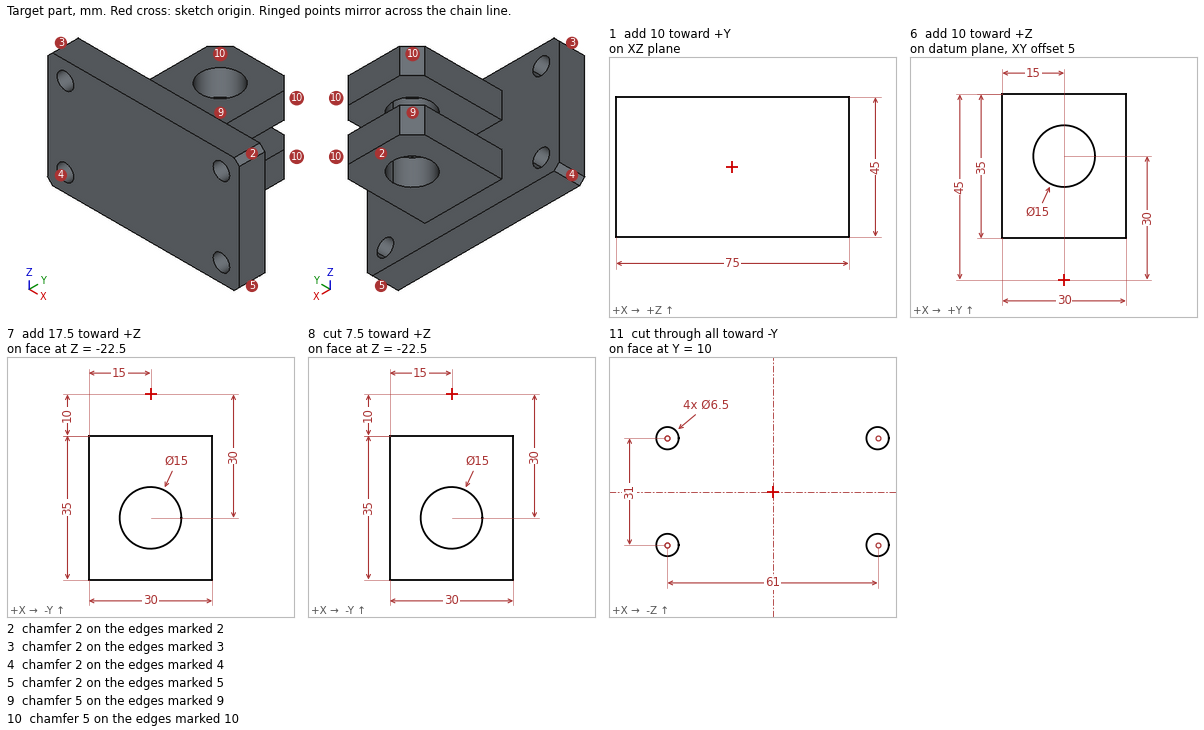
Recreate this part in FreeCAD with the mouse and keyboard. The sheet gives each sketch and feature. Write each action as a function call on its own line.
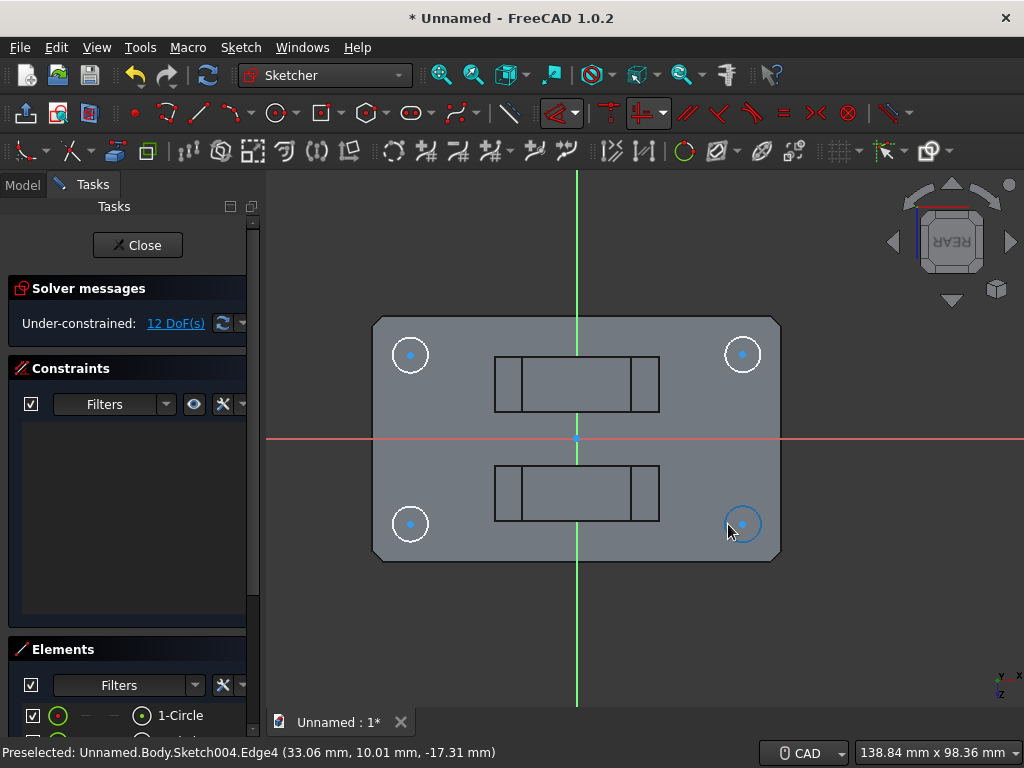
click(423, 343)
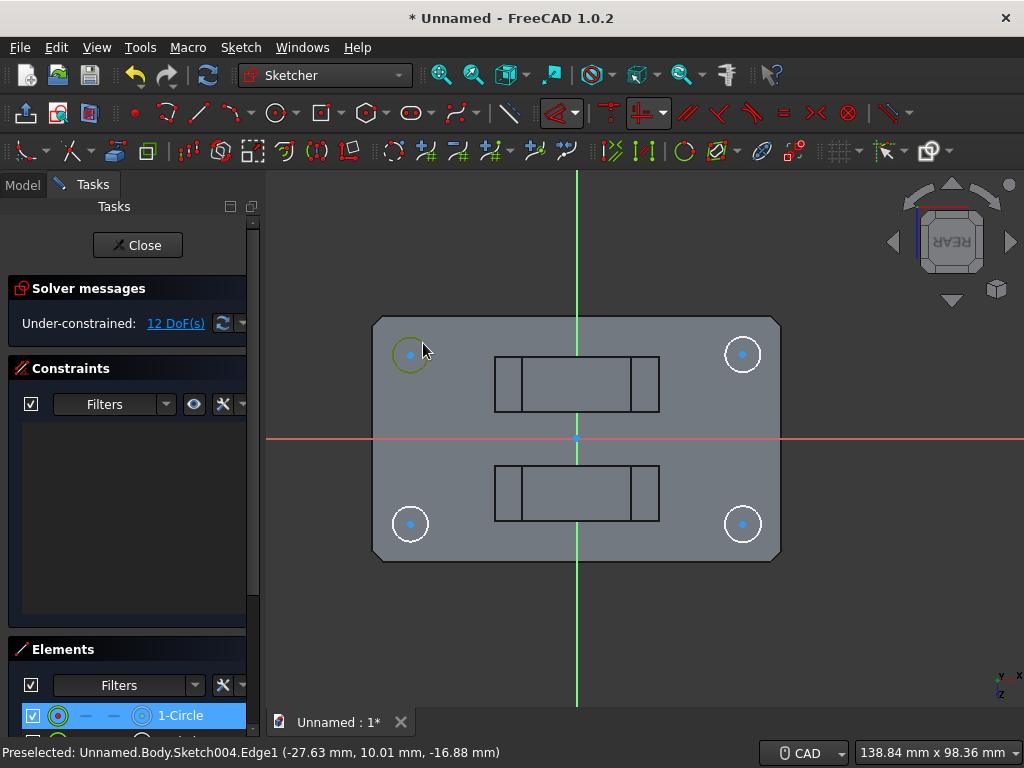
click(423, 512)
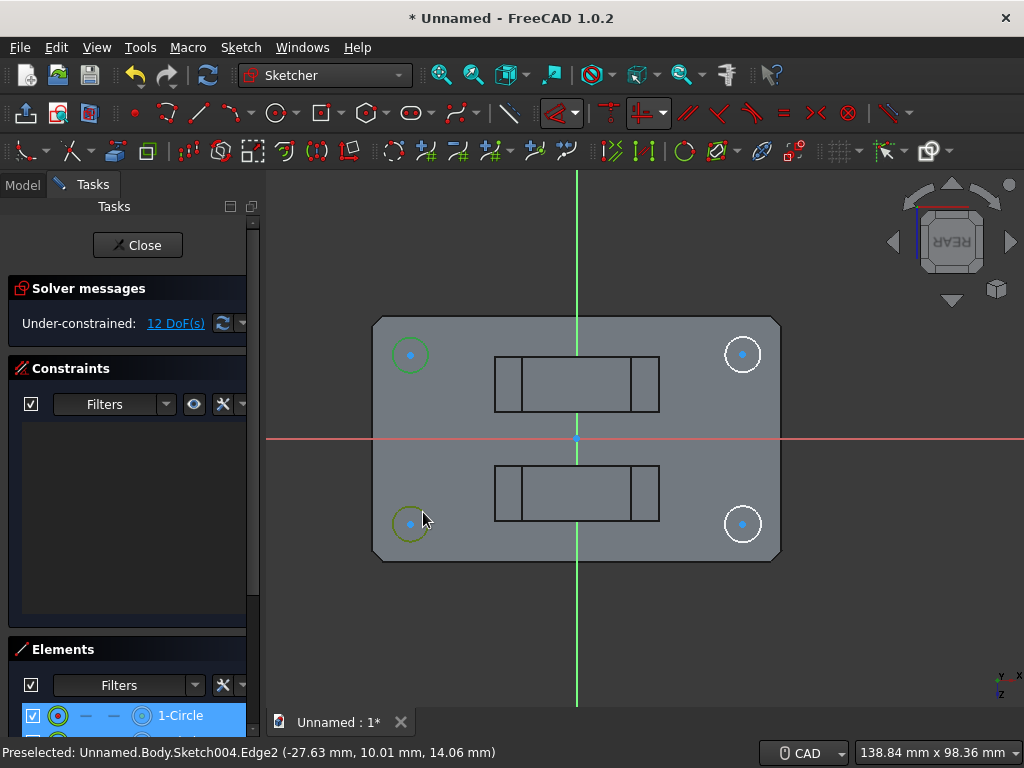
click(756, 511)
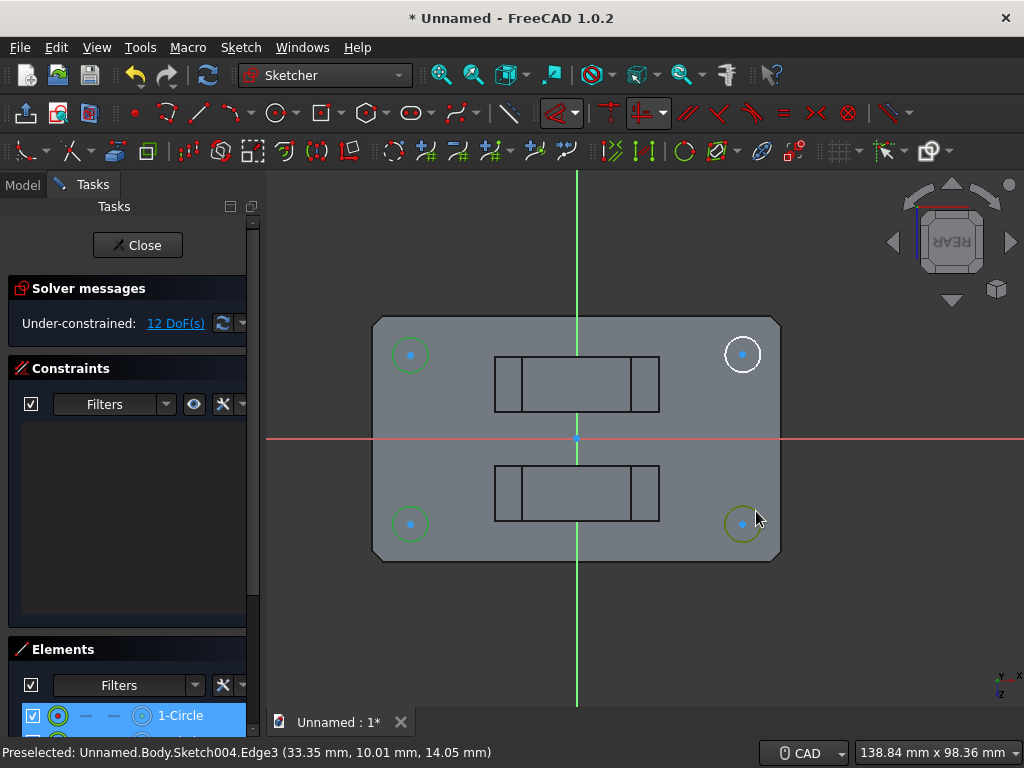
click(755, 342)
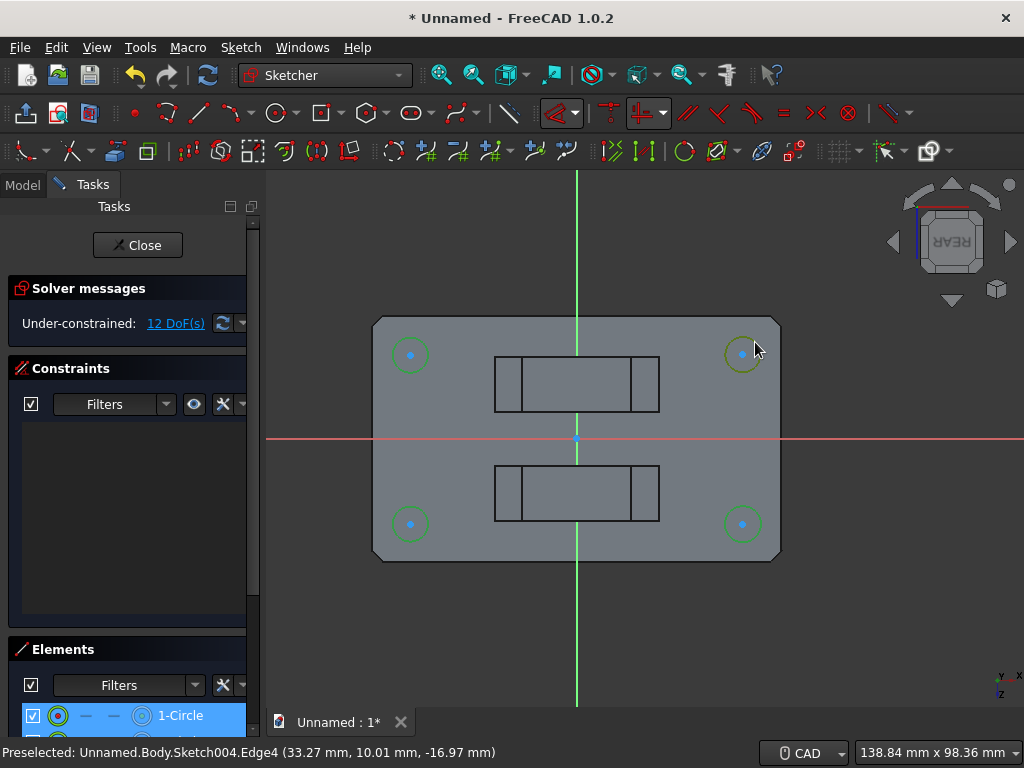
key(e)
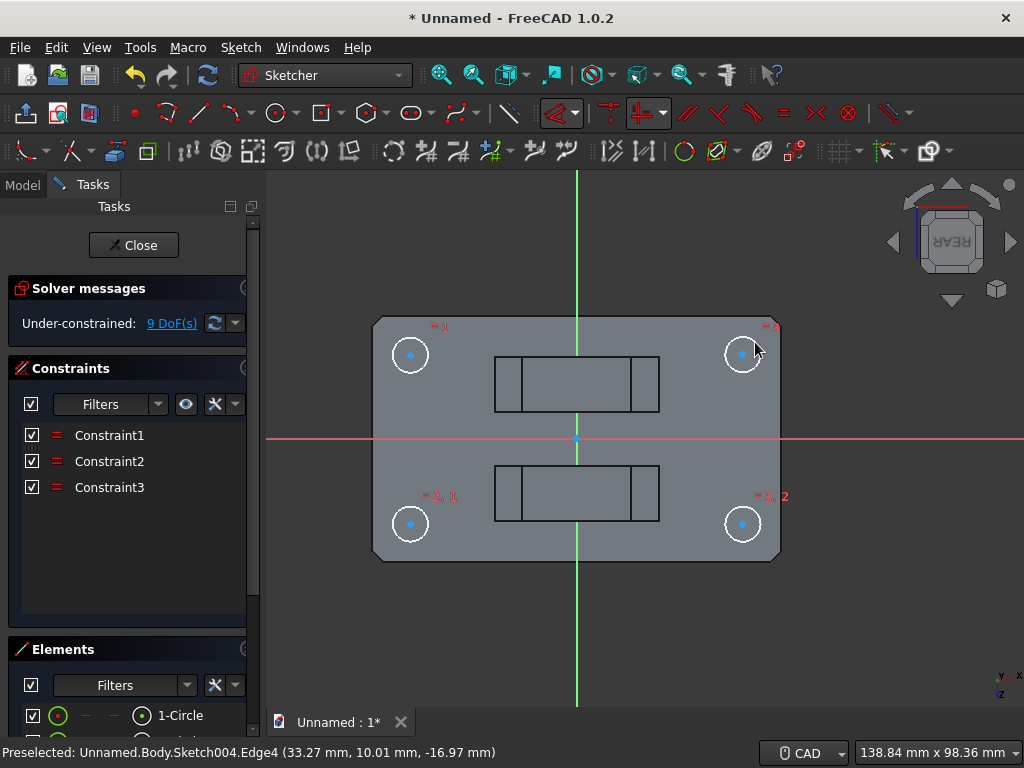
click(410, 355)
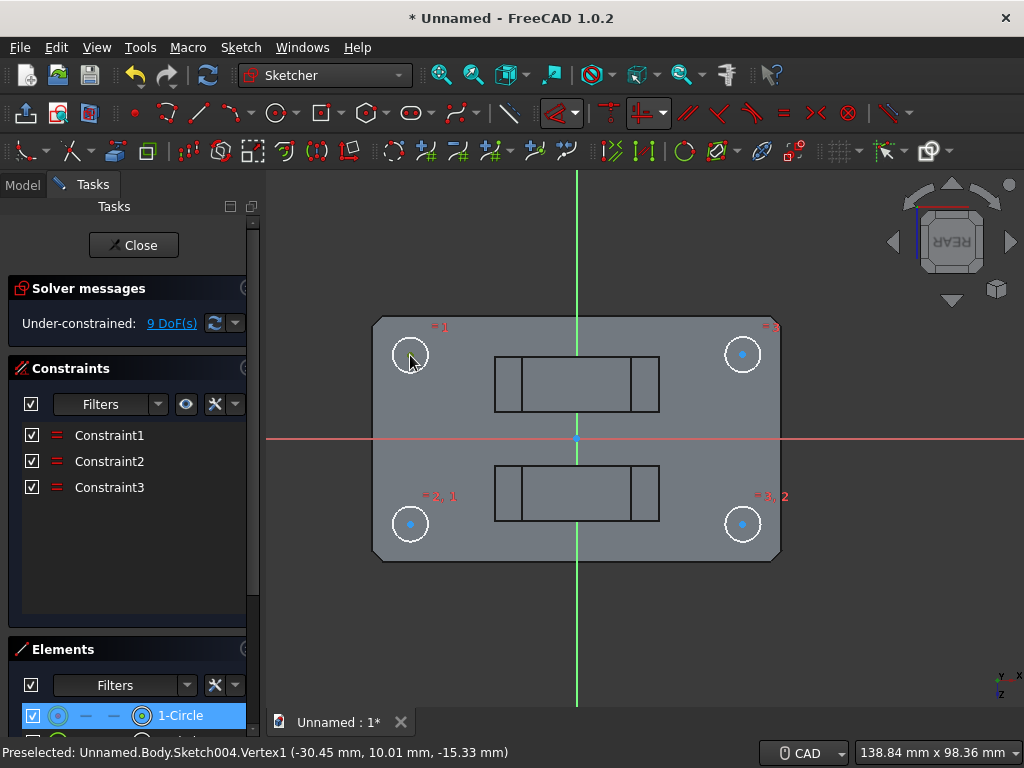
click(410, 524)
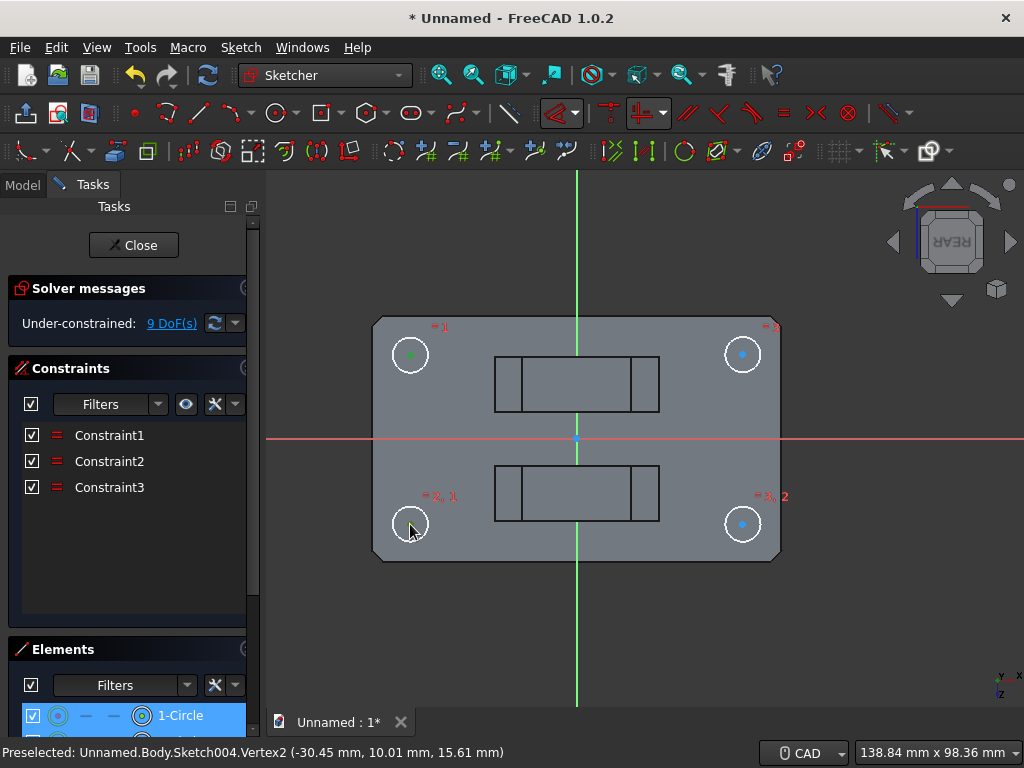
click(334, 439)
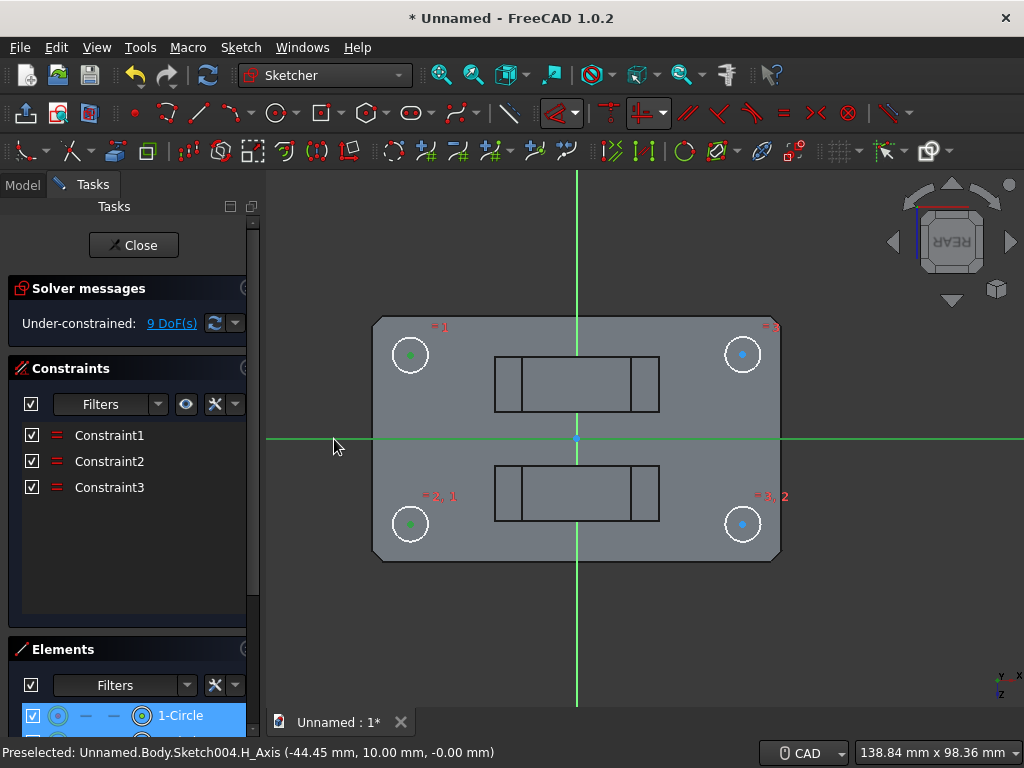
key(s)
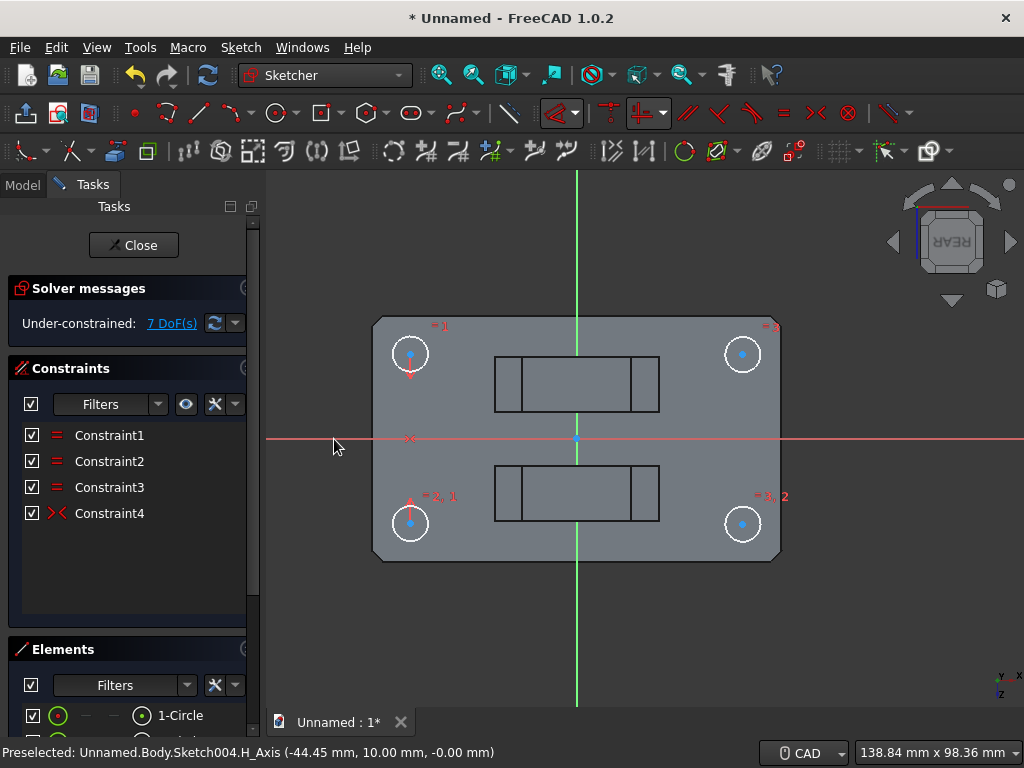
click(410, 524)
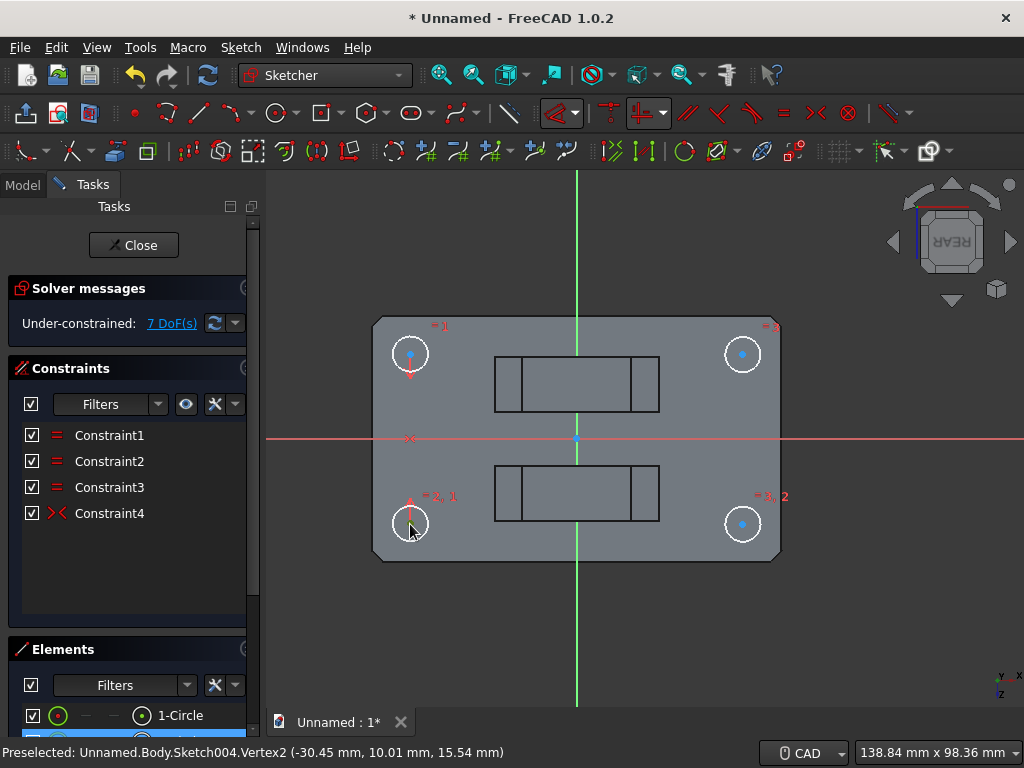
click(743, 524)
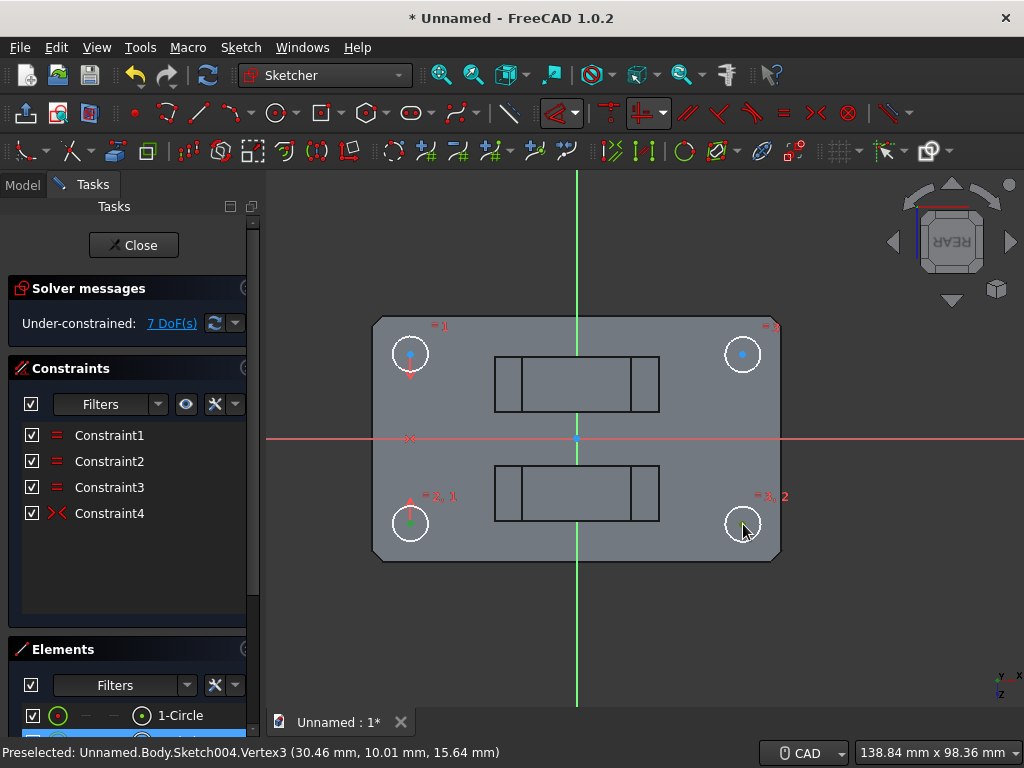
click(577, 645)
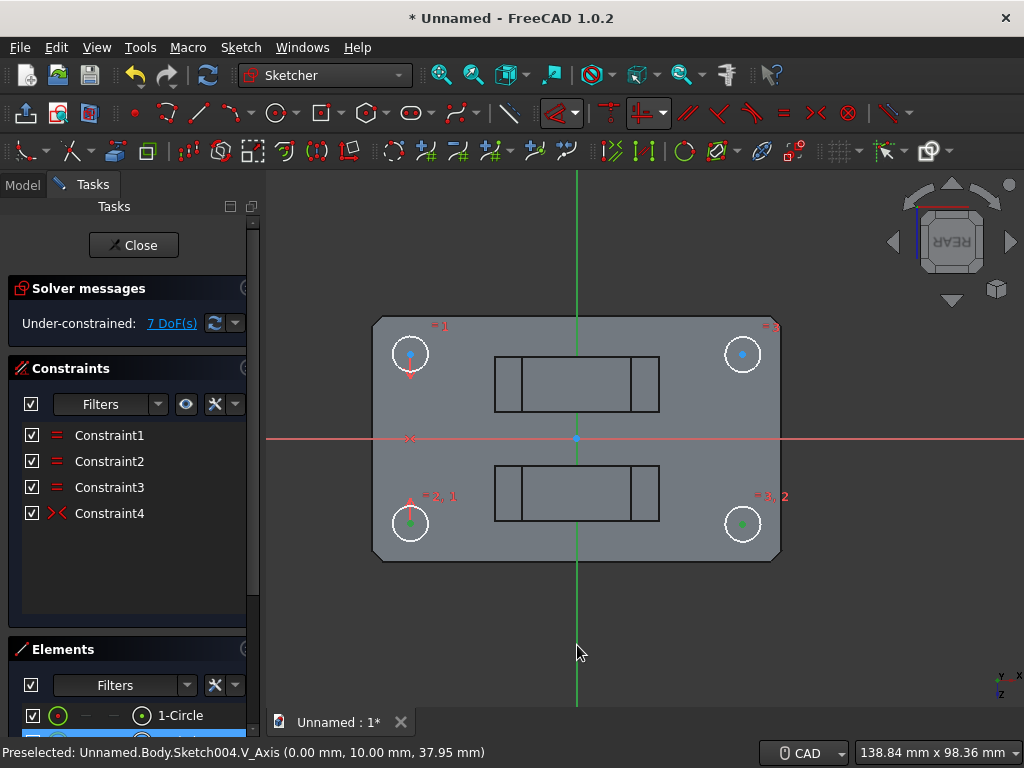
key(s)